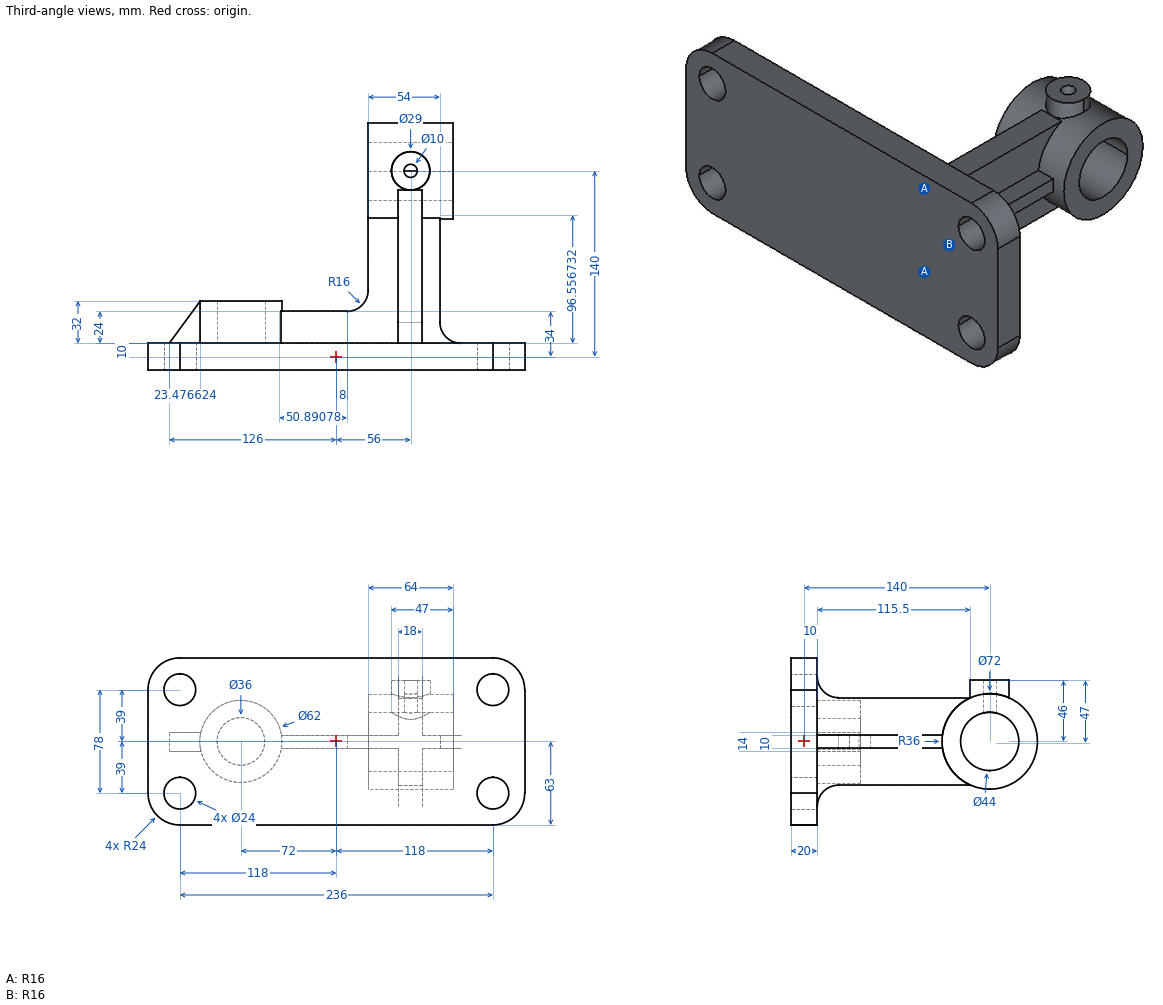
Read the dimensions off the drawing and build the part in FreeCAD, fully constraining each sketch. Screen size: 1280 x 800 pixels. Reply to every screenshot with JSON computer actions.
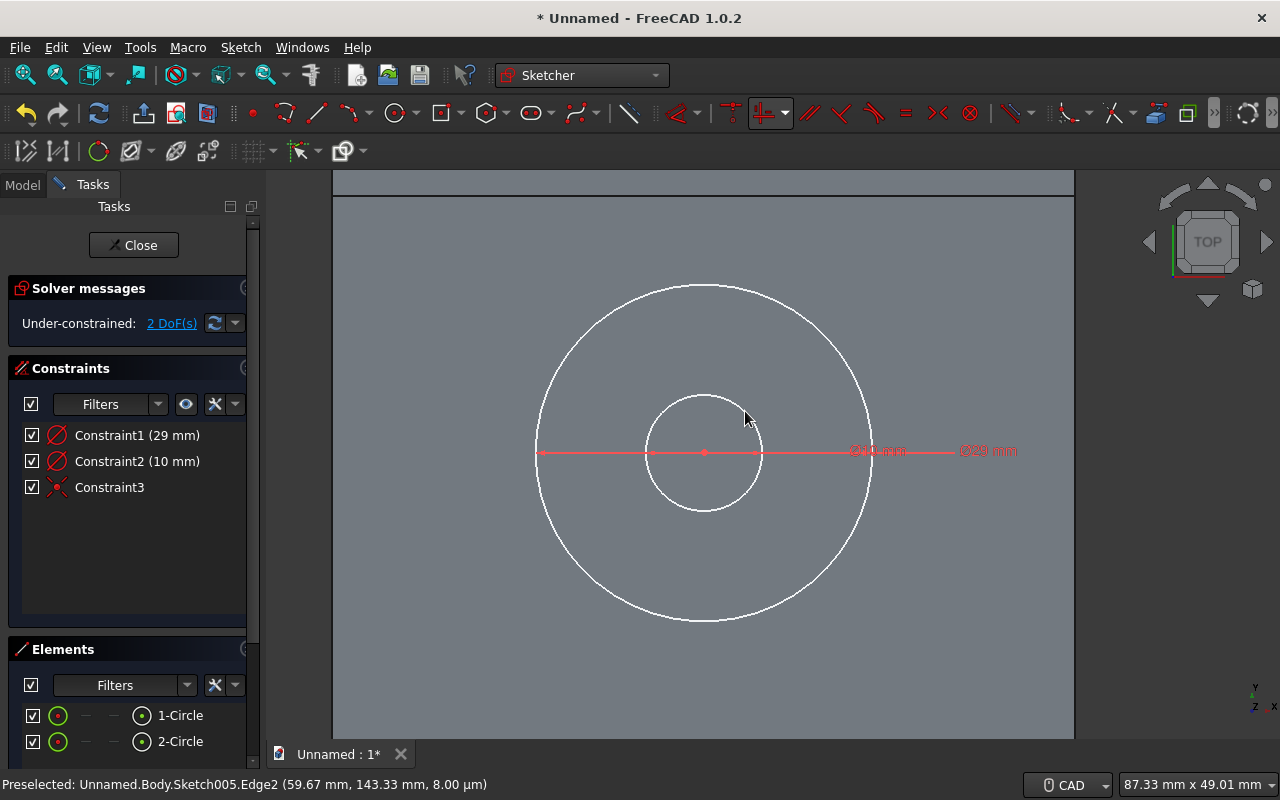
{"action": "left_click", "coordinate": [676, 114]}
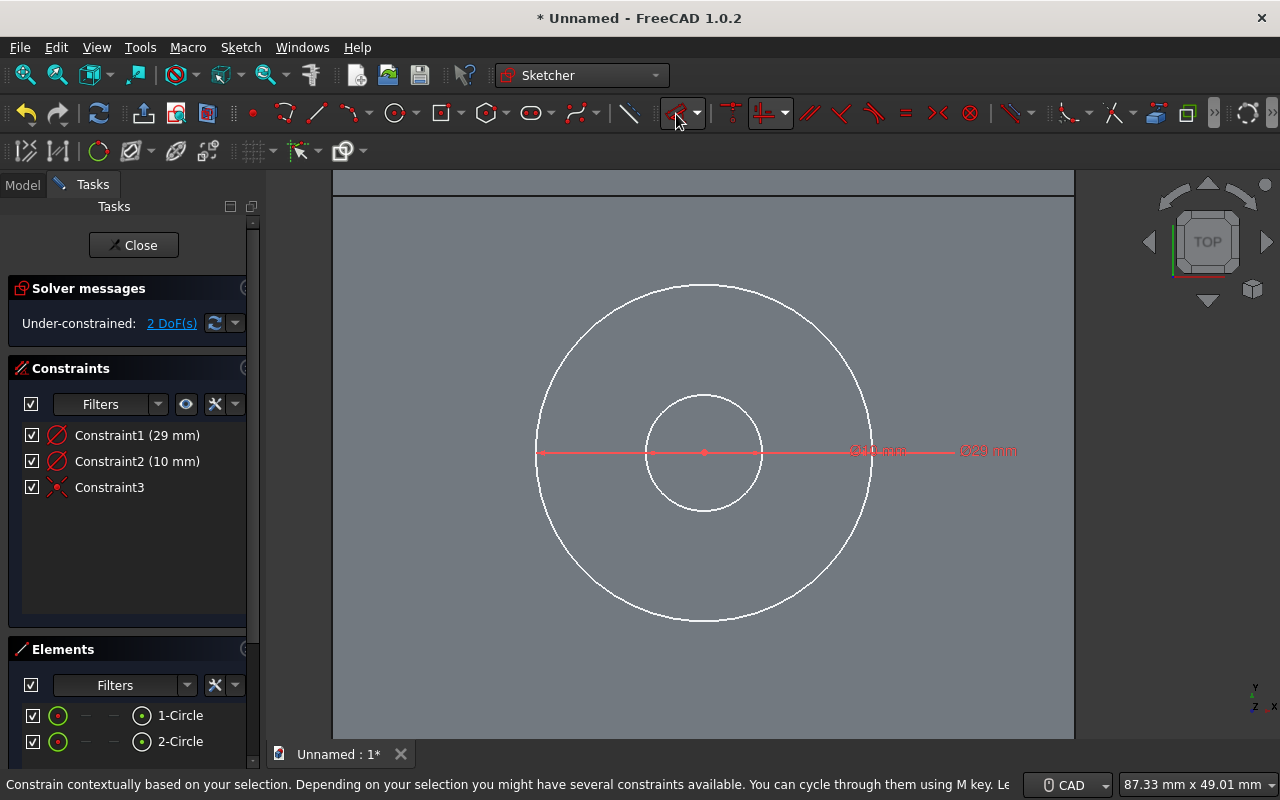
{"action": "left_click", "coordinate": [704, 453]}
{"action": "left_click", "coordinate": [499, 419]}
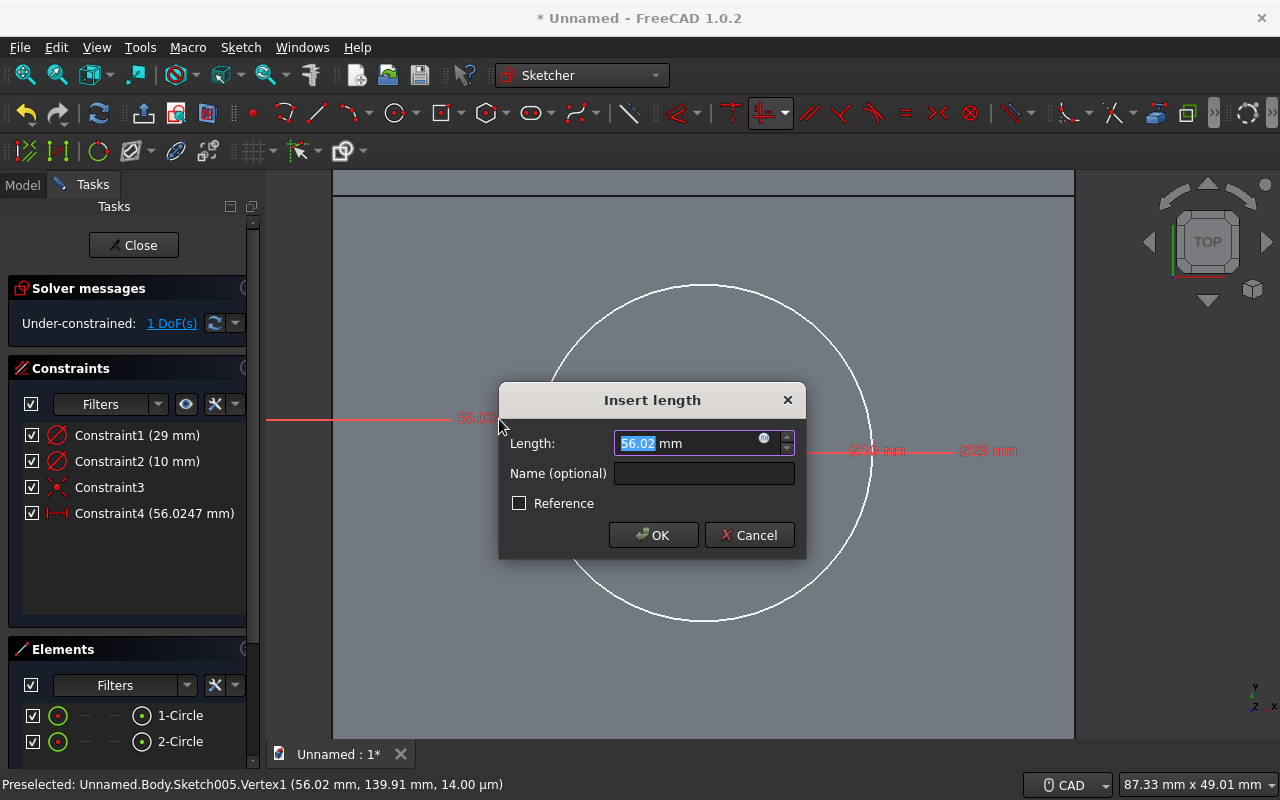
{"action": "type", "text": "56"}
{"action": "key", "text": "Return"}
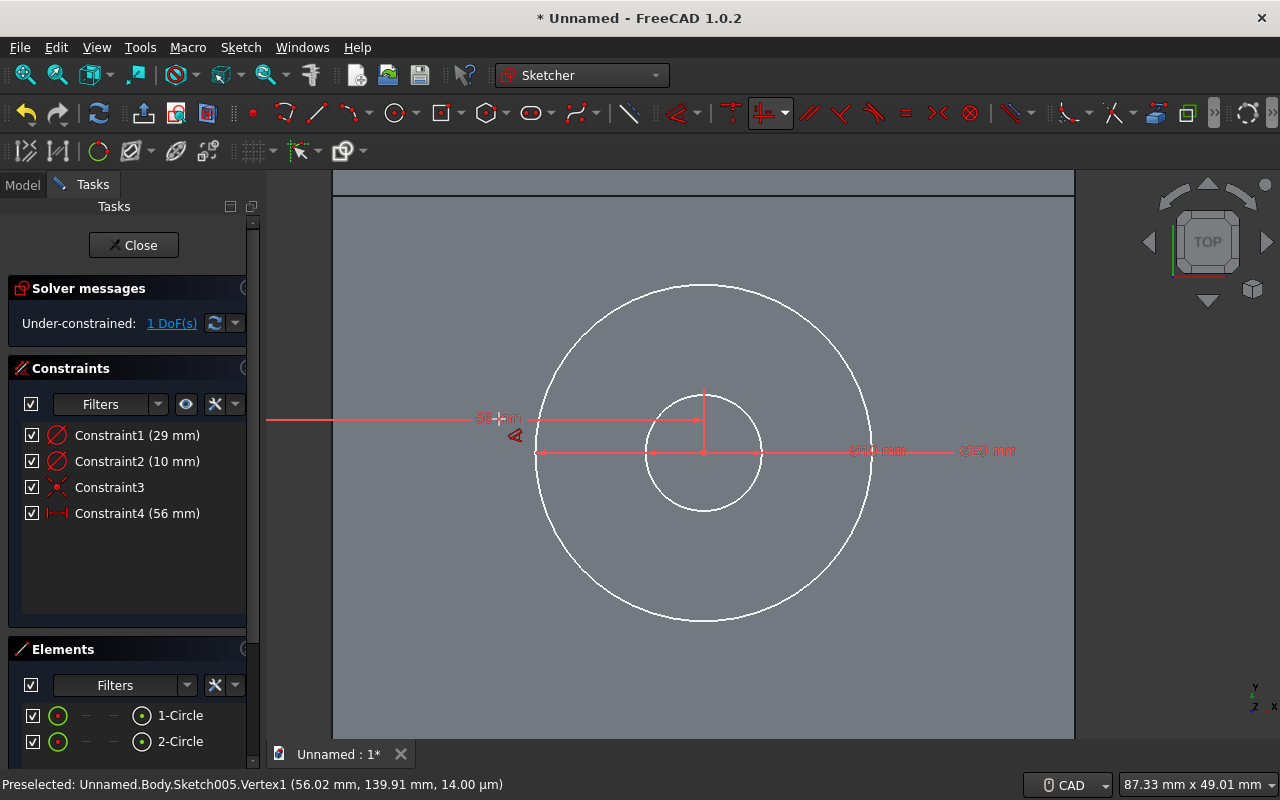
{"action": "left_click", "coordinate": [704, 453]}
{"action": "left_click", "coordinate": [738, 582]}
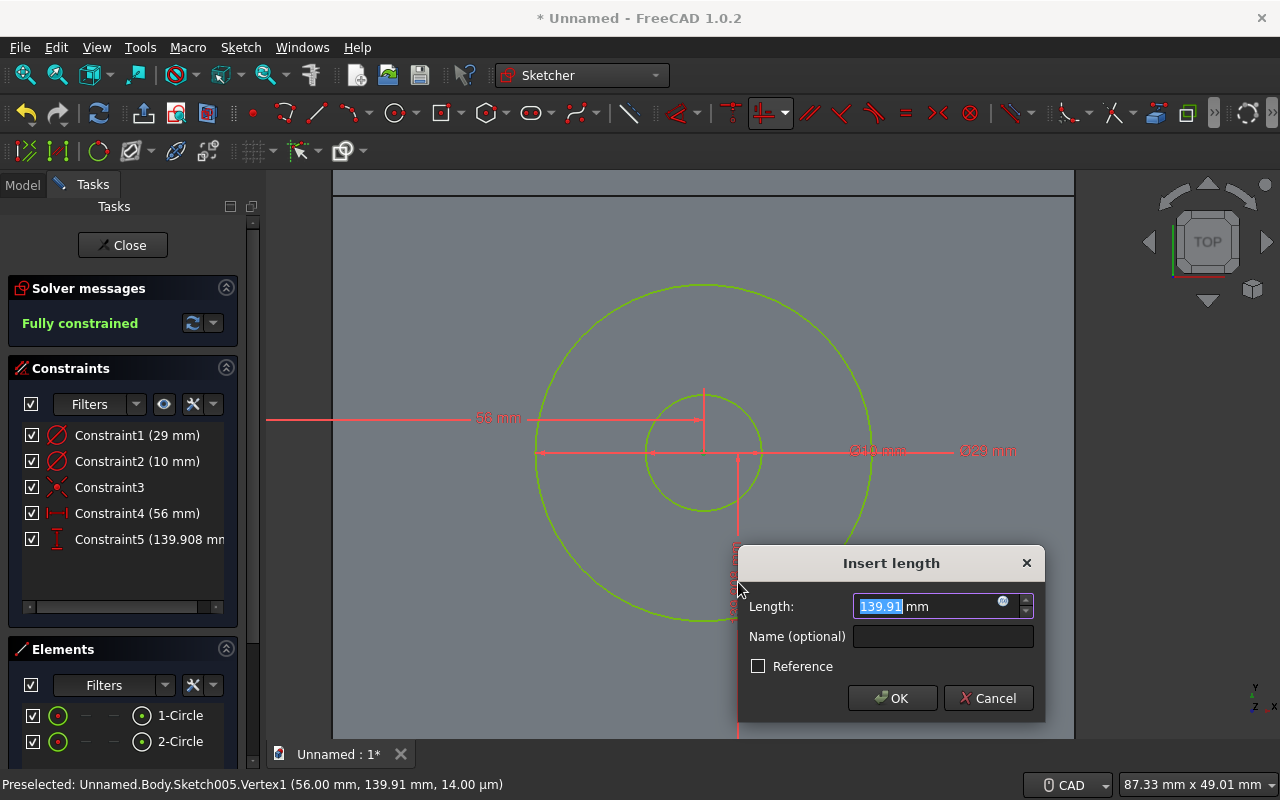
{"action": "type", "text": "140"}
{"action": "key", "text": "Return"}
{"action": "key", "text": "Escape"}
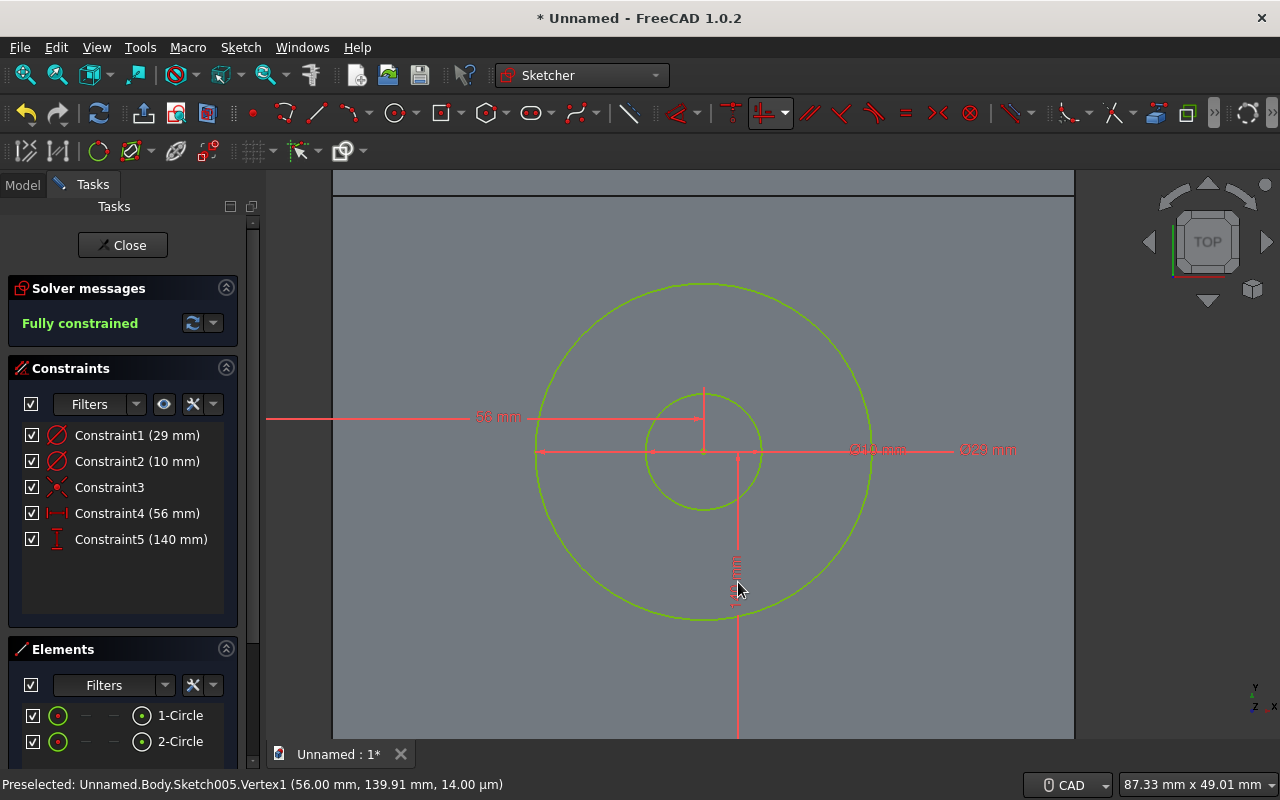
{"action": "left_click", "coordinate": [123, 245]}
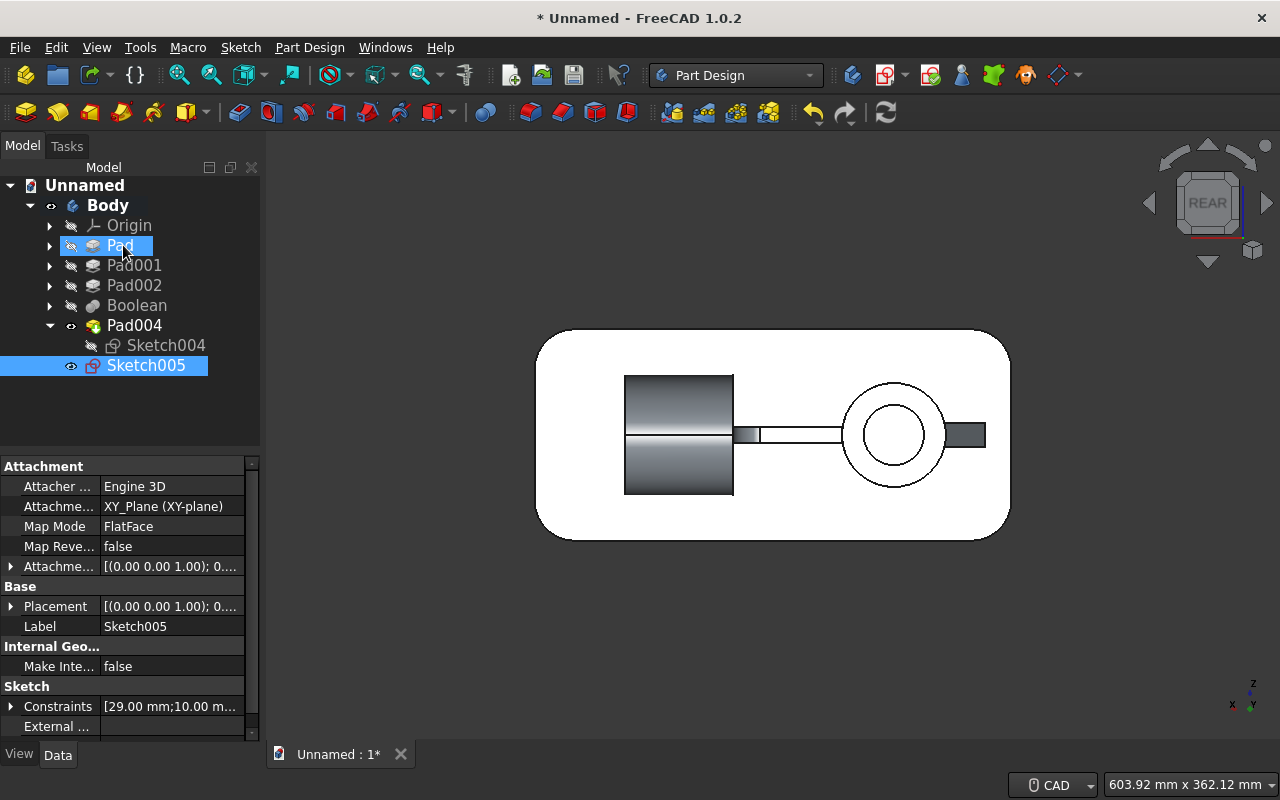
{"action": "left_click", "coordinate": [26, 112]}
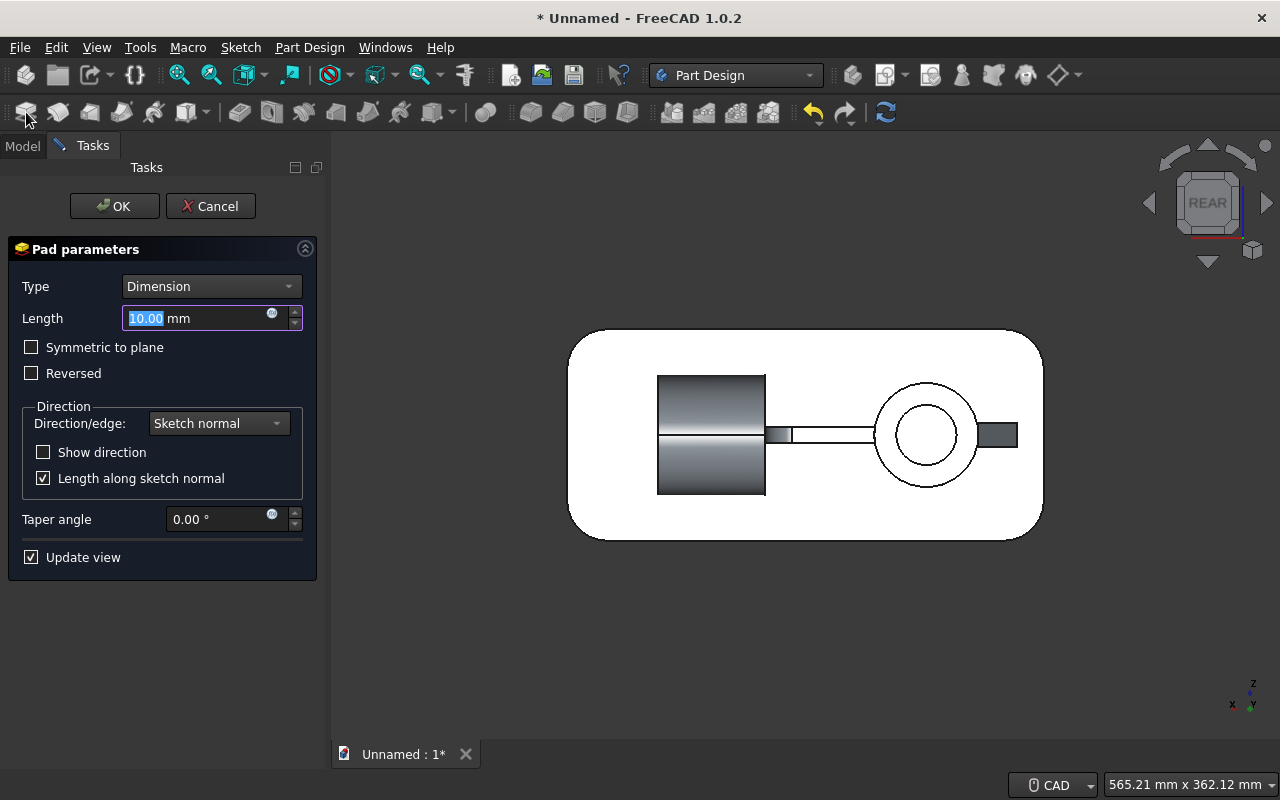
{"action": "type", "text": "46"}
{"action": "key", "text": "Tab"}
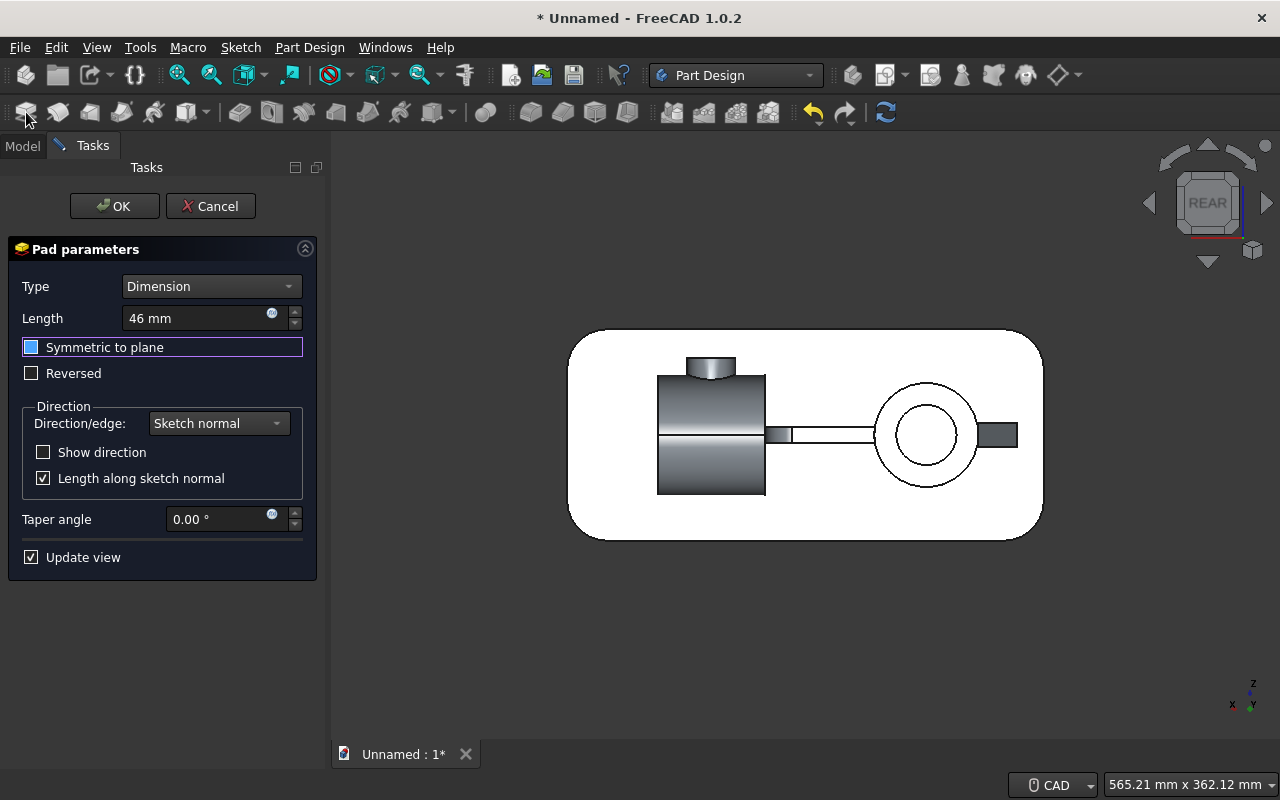
{"action": "left_click", "coordinate": [115, 206]}